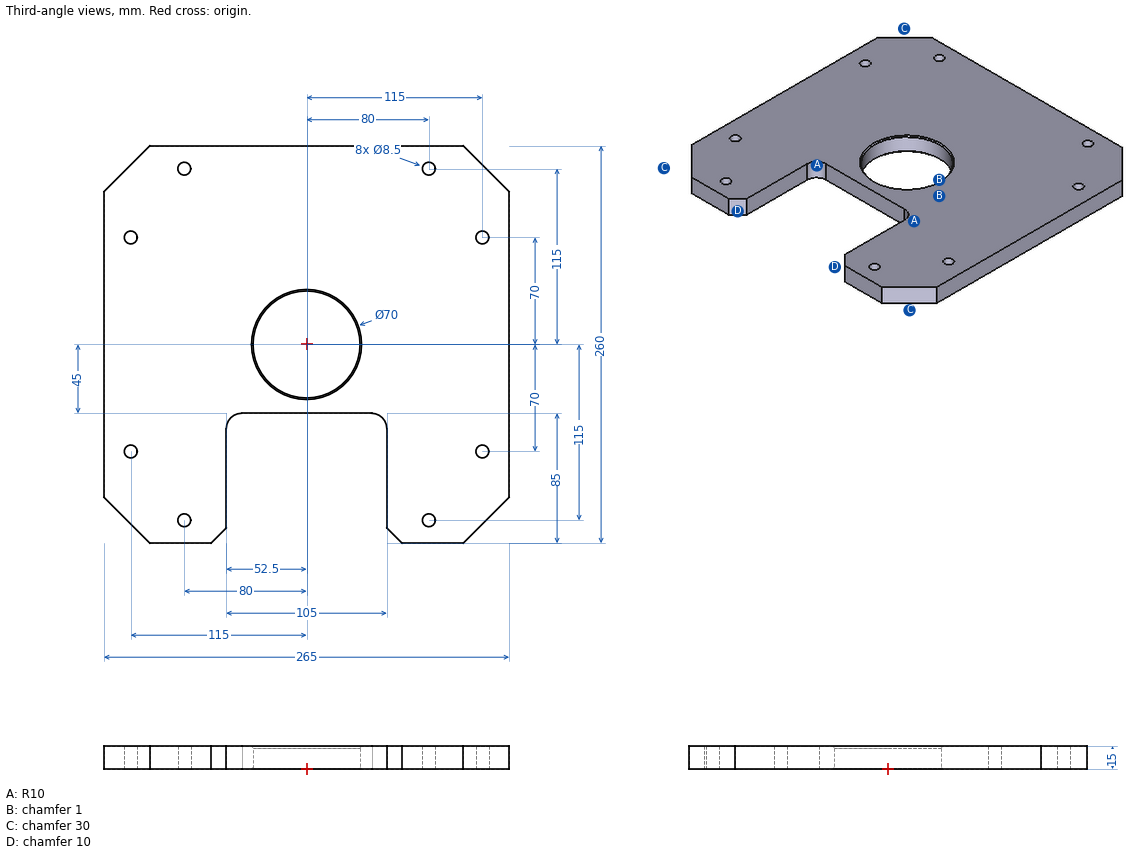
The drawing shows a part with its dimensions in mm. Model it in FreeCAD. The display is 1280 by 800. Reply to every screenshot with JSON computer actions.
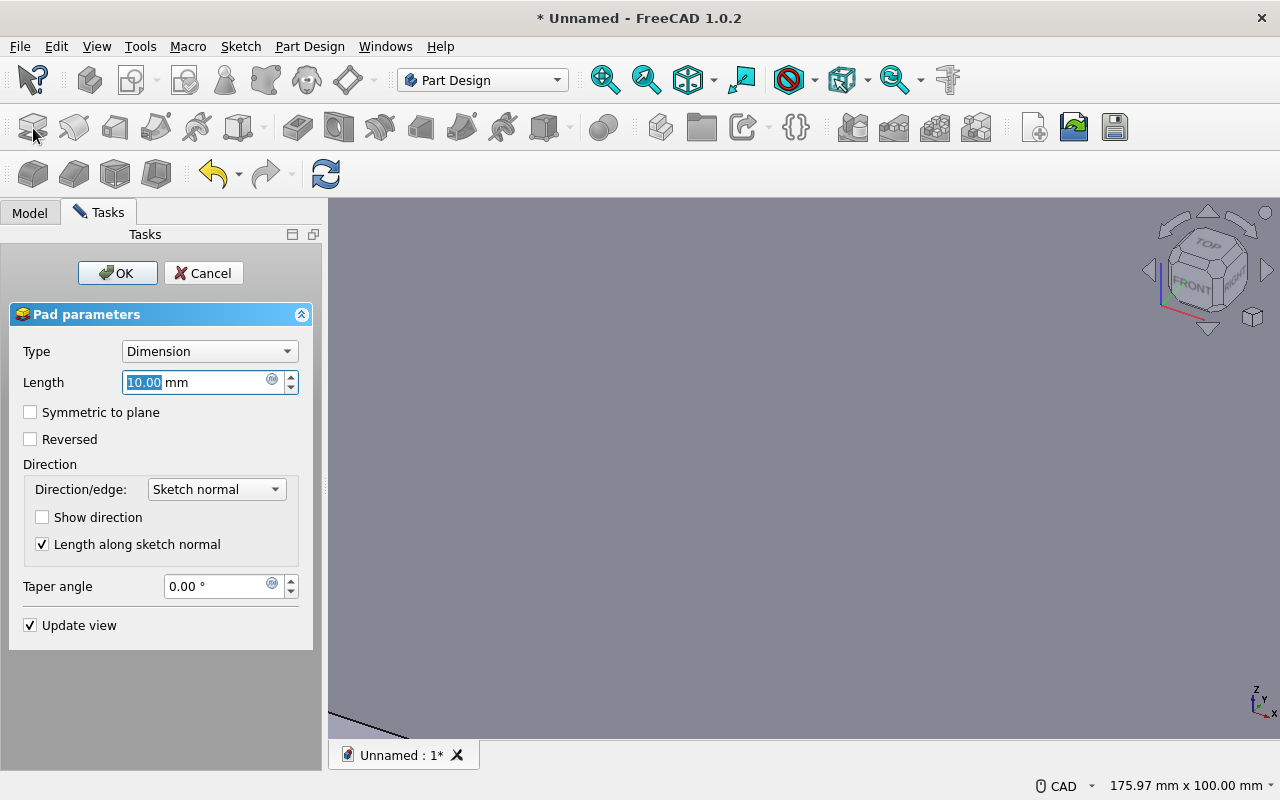
{"action": "type", "text": "15"}
{"action": "key", "text": "Tab"}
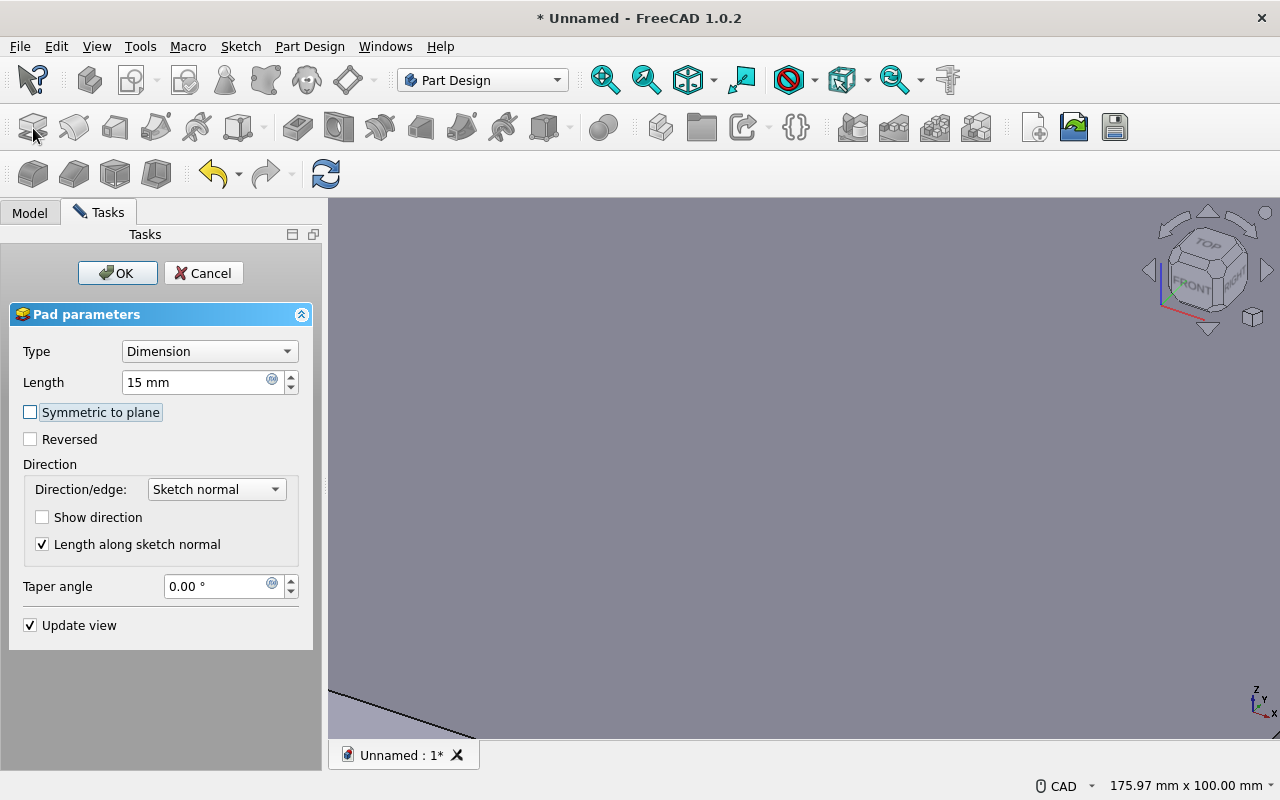
{"action": "left_click", "coordinate": [118, 273]}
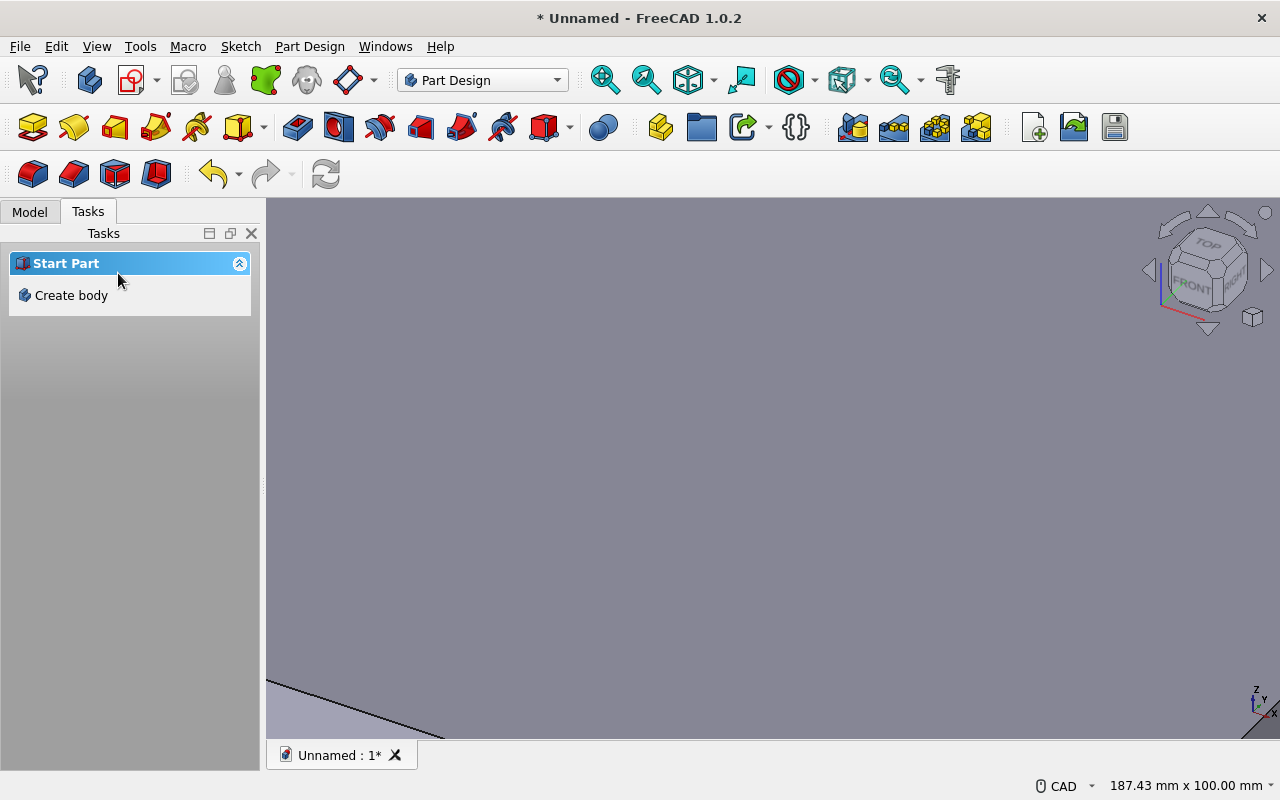
{"action": "left_click", "coordinate": [606, 80]}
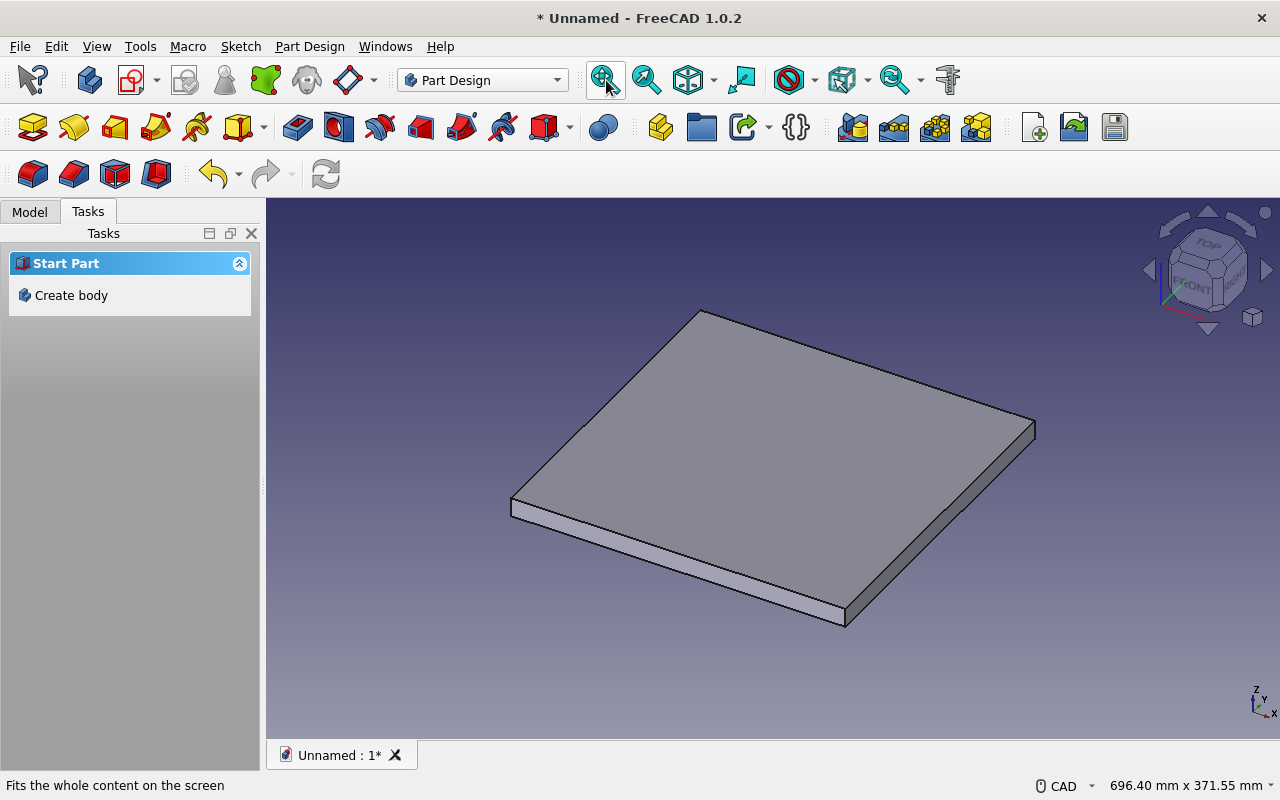
{"action": "key", "text": "5"}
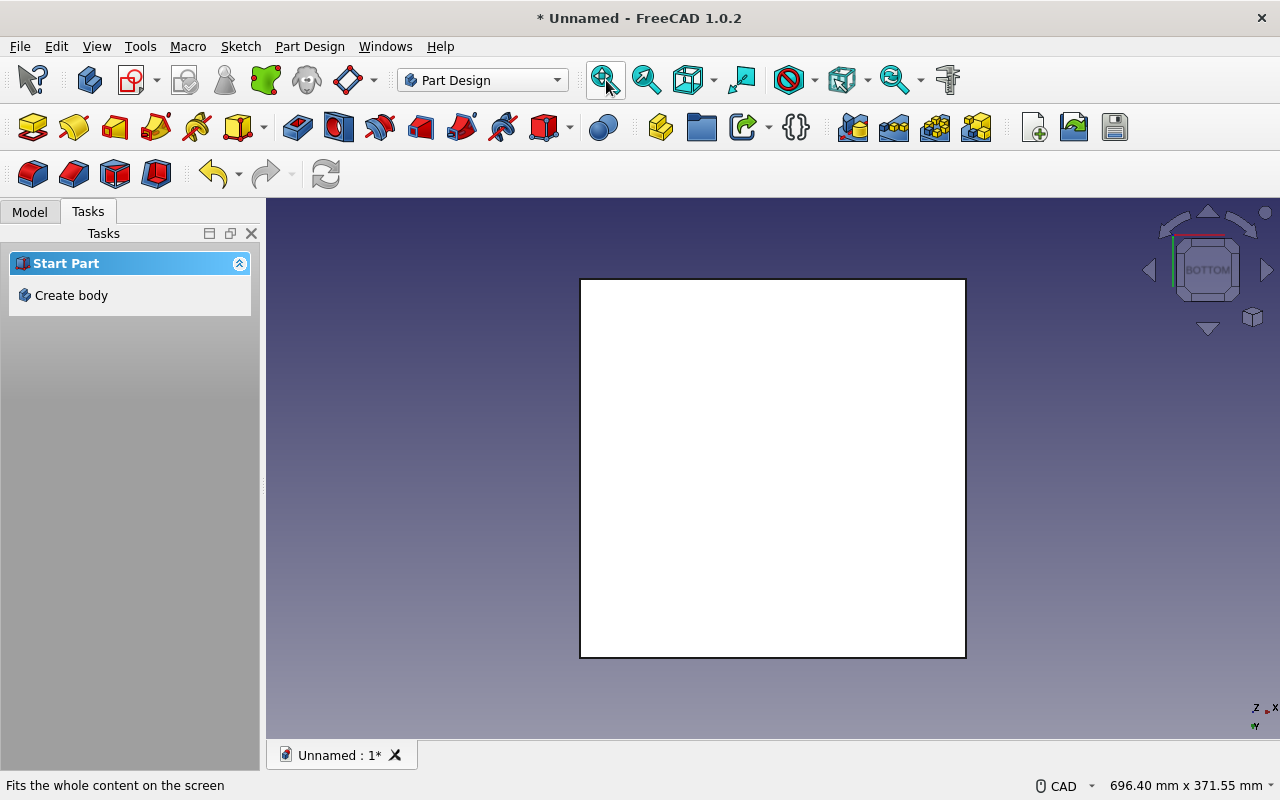
{"action": "left_click", "coordinate": [773, 467]}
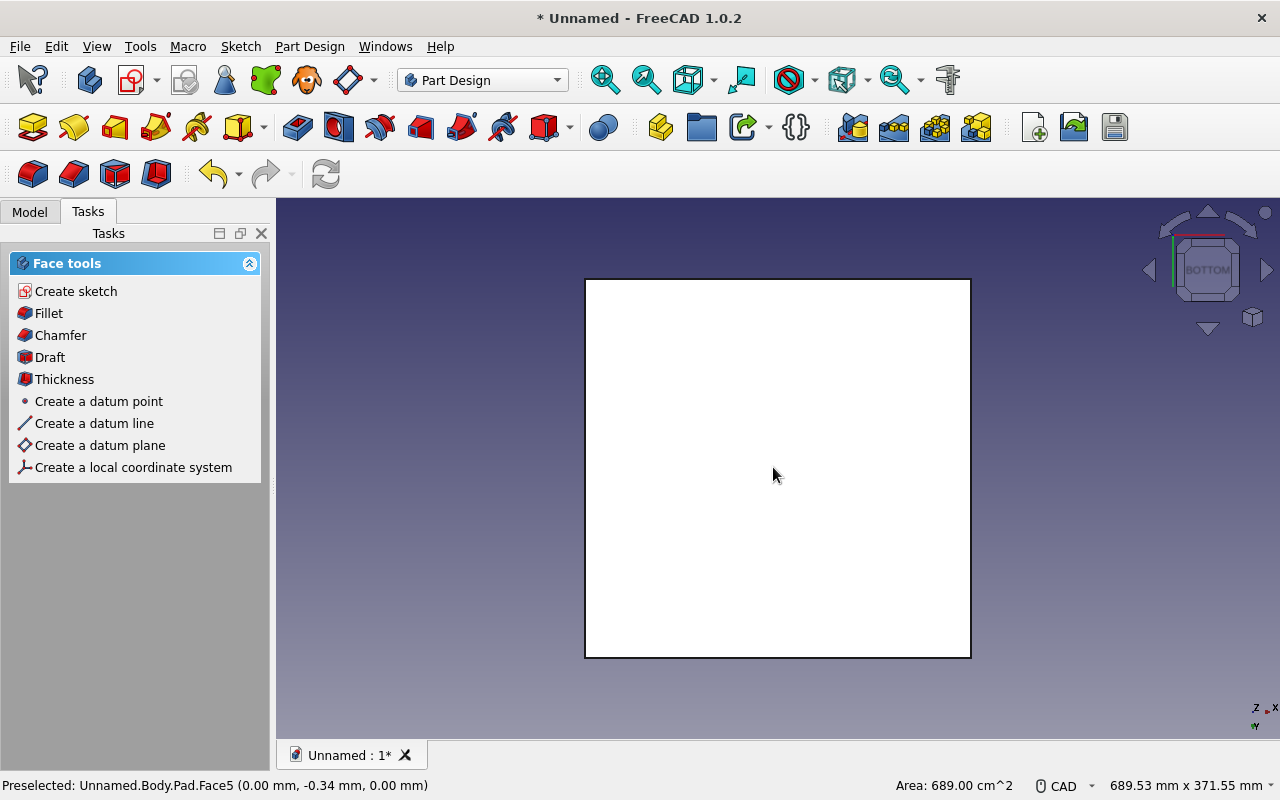
{"action": "left_click", "coordinate": [130, 80]}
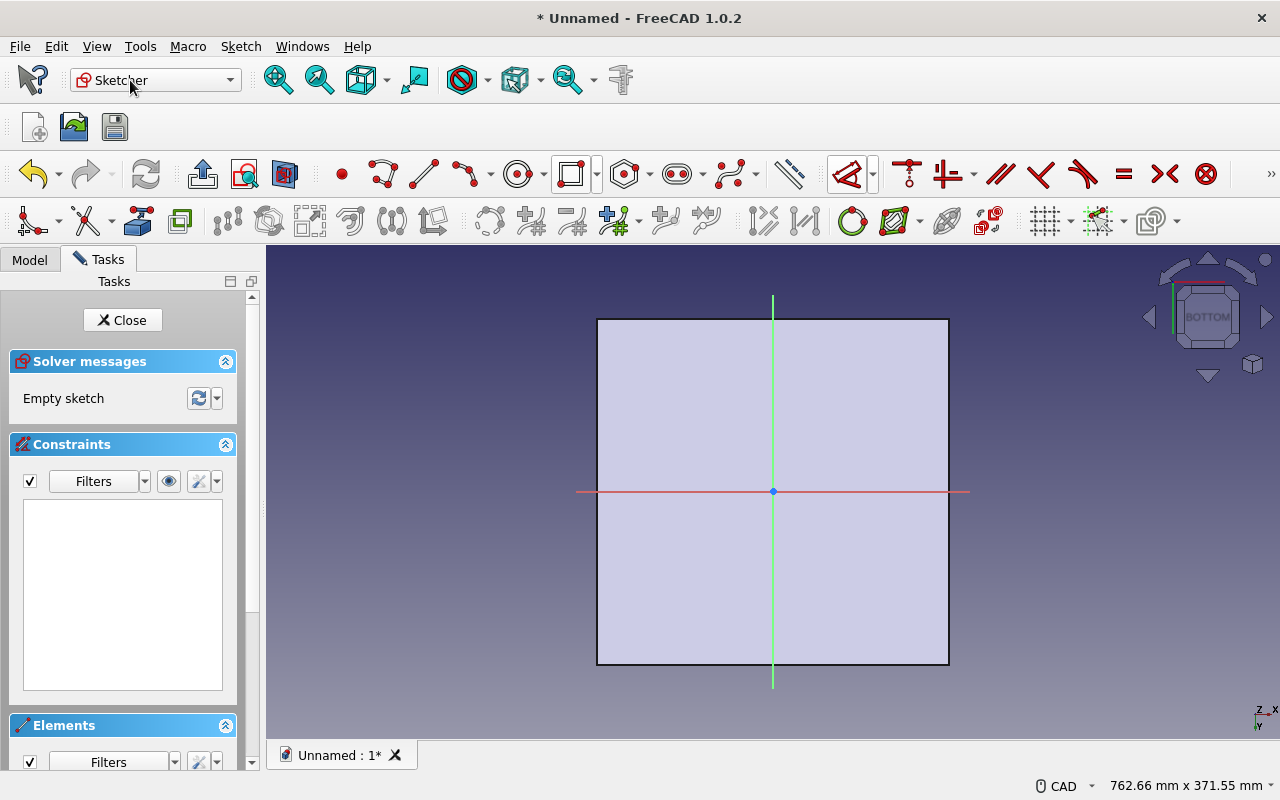
{"action": "left_click", "coordinate": [518, 174]}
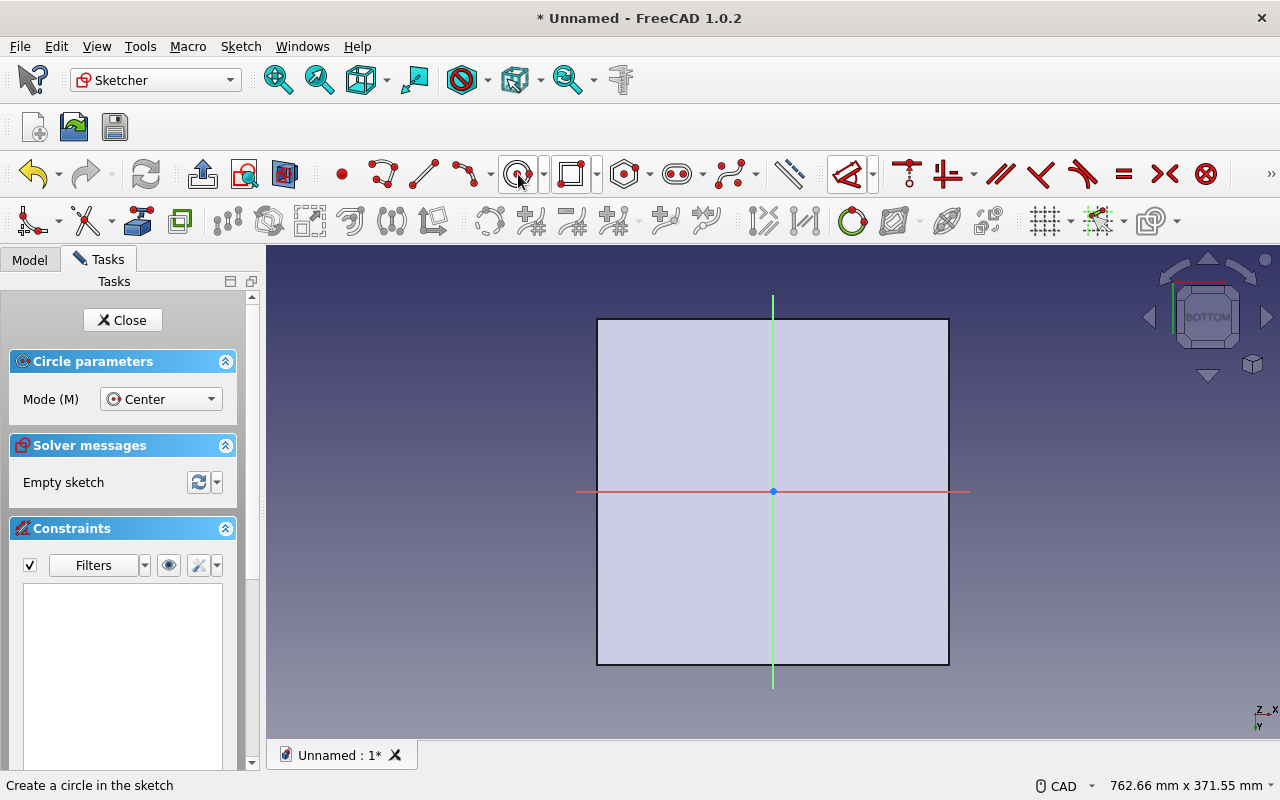
{"action": "scroll", "coordinate": [879, 645], "scroll_direction": "up", "scroll_amount": 7}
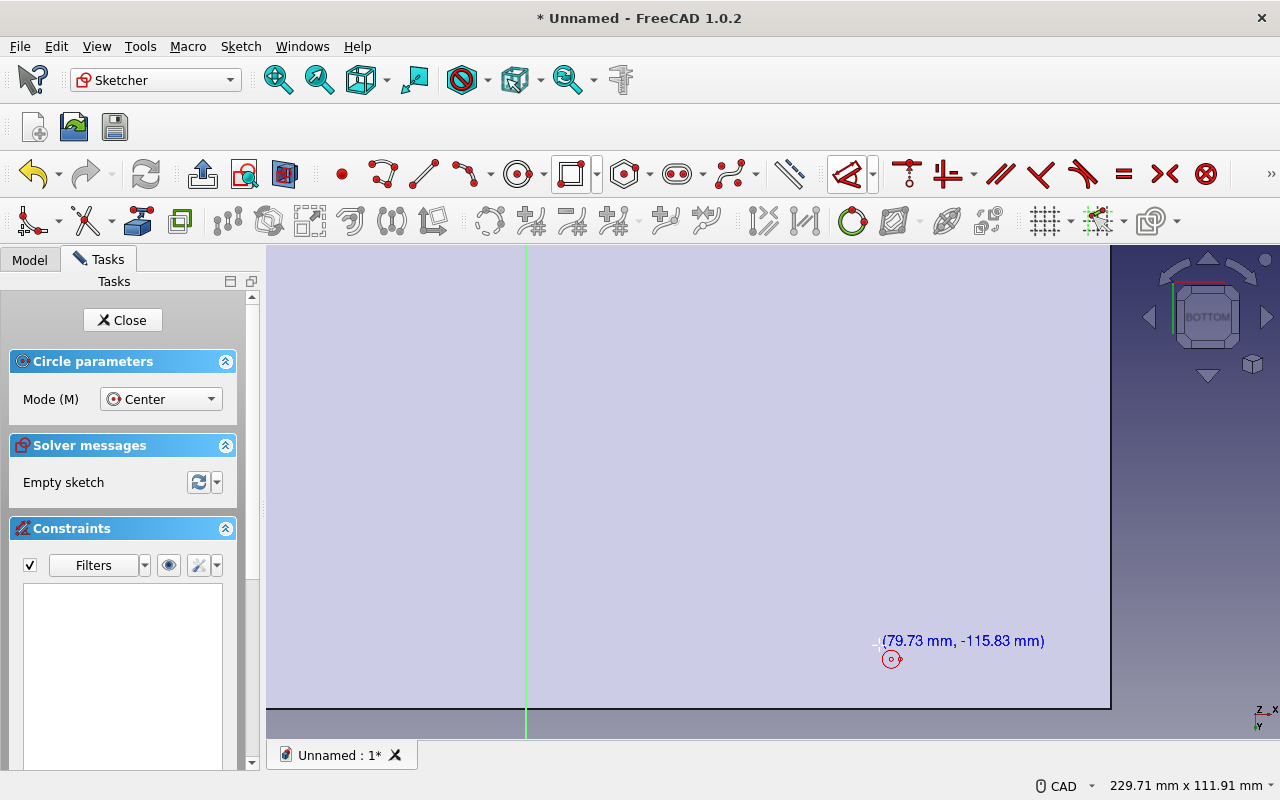
{"action": "scroll", "coordinate": [789, 646], "scroll_direction": "down", "scroll_amount": 7}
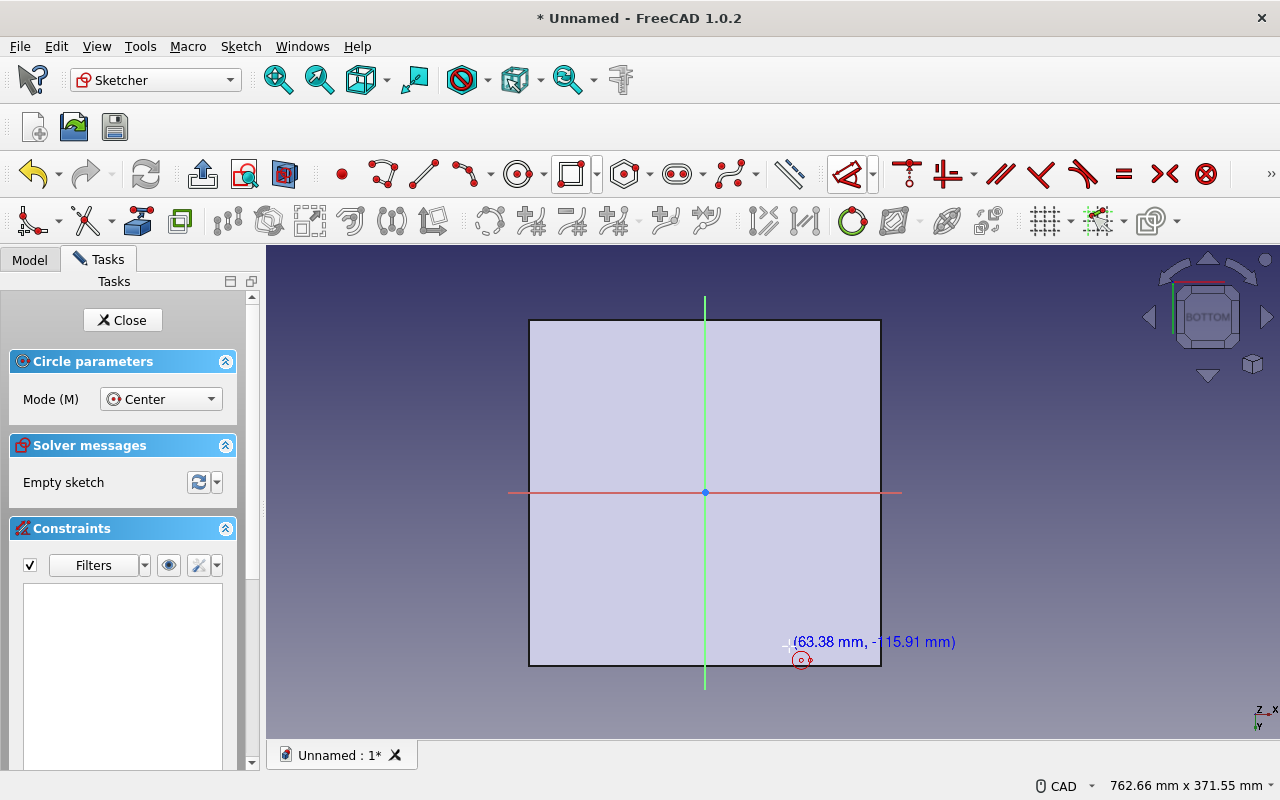
{"action": "left_click", "coordinate": [811, 646]}
{"action": "mouse_move", "coordinate": [815, 642]}